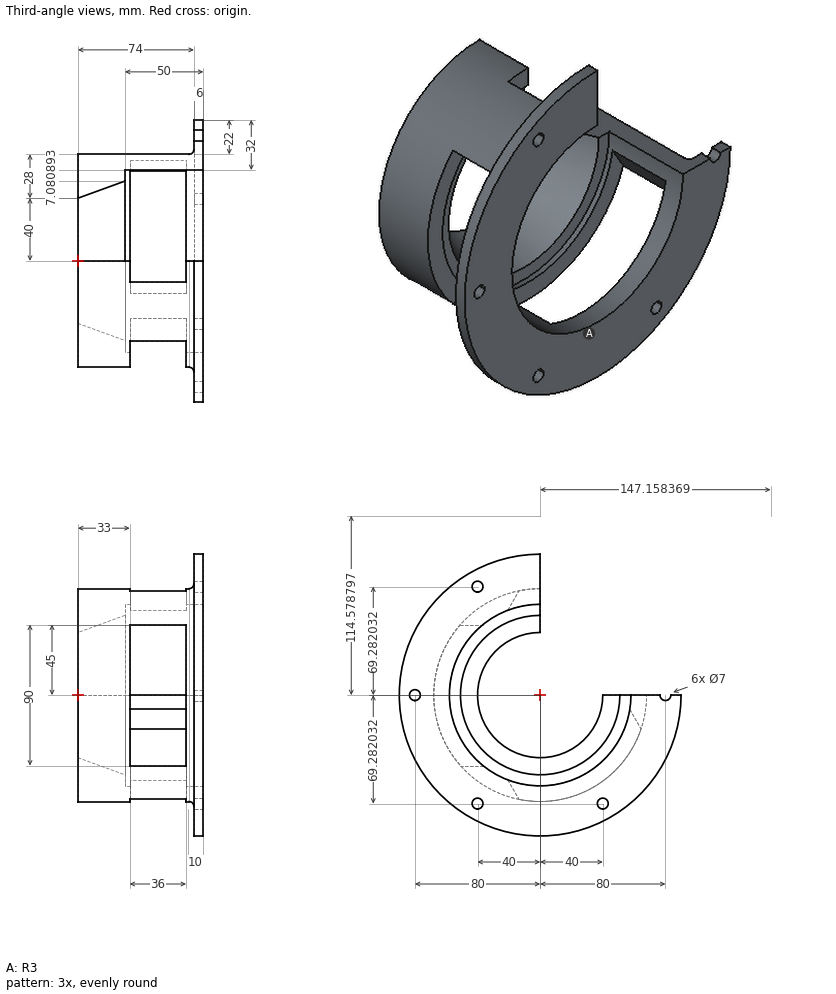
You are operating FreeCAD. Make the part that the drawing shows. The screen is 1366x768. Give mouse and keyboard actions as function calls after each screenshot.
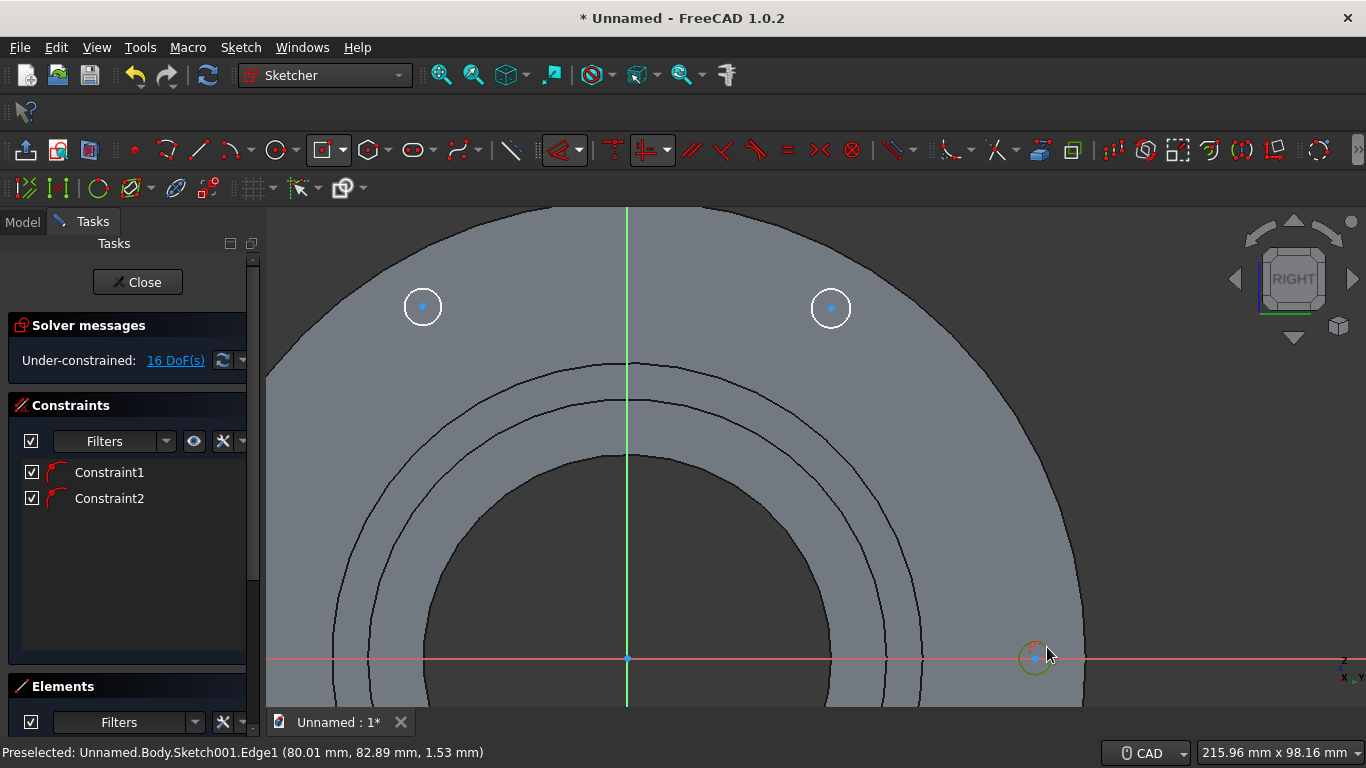
scroll(846, 293, down, 4)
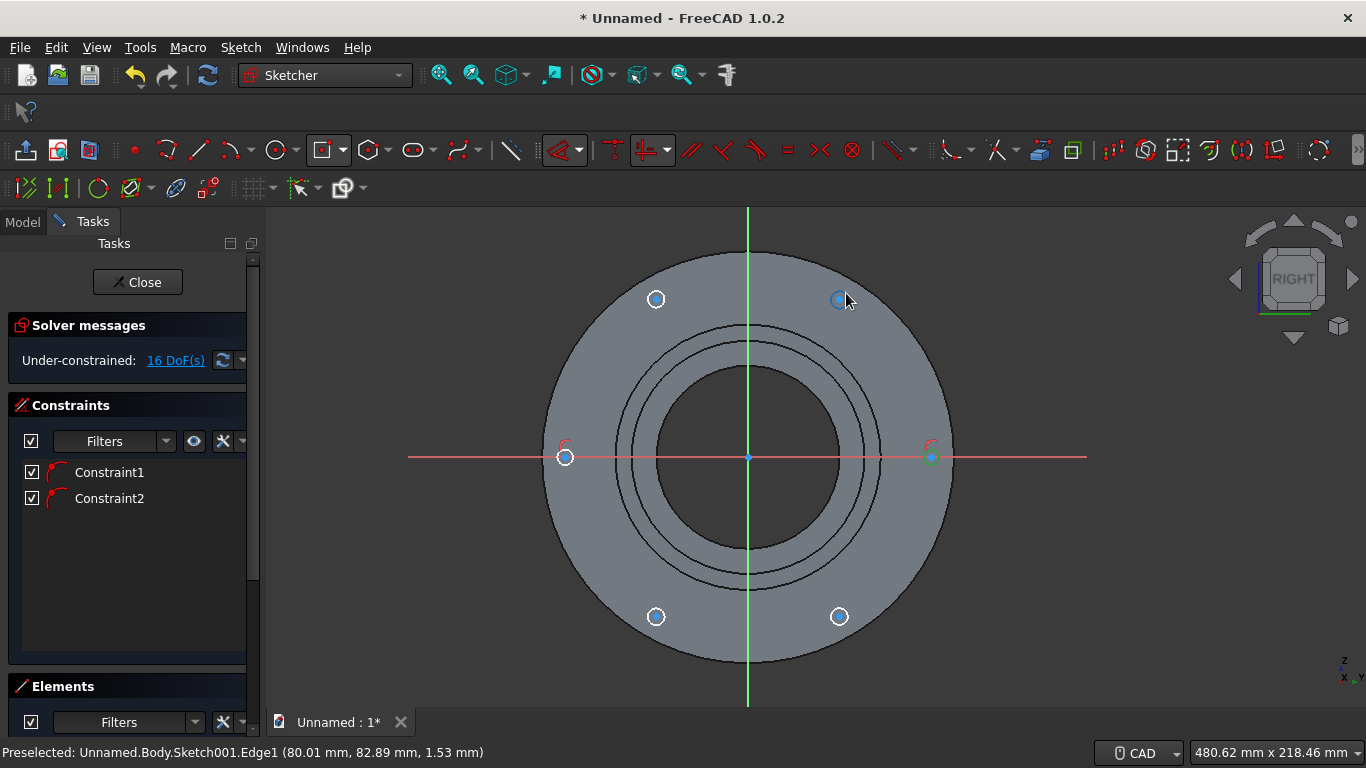
scroll(845, 611, up, 3)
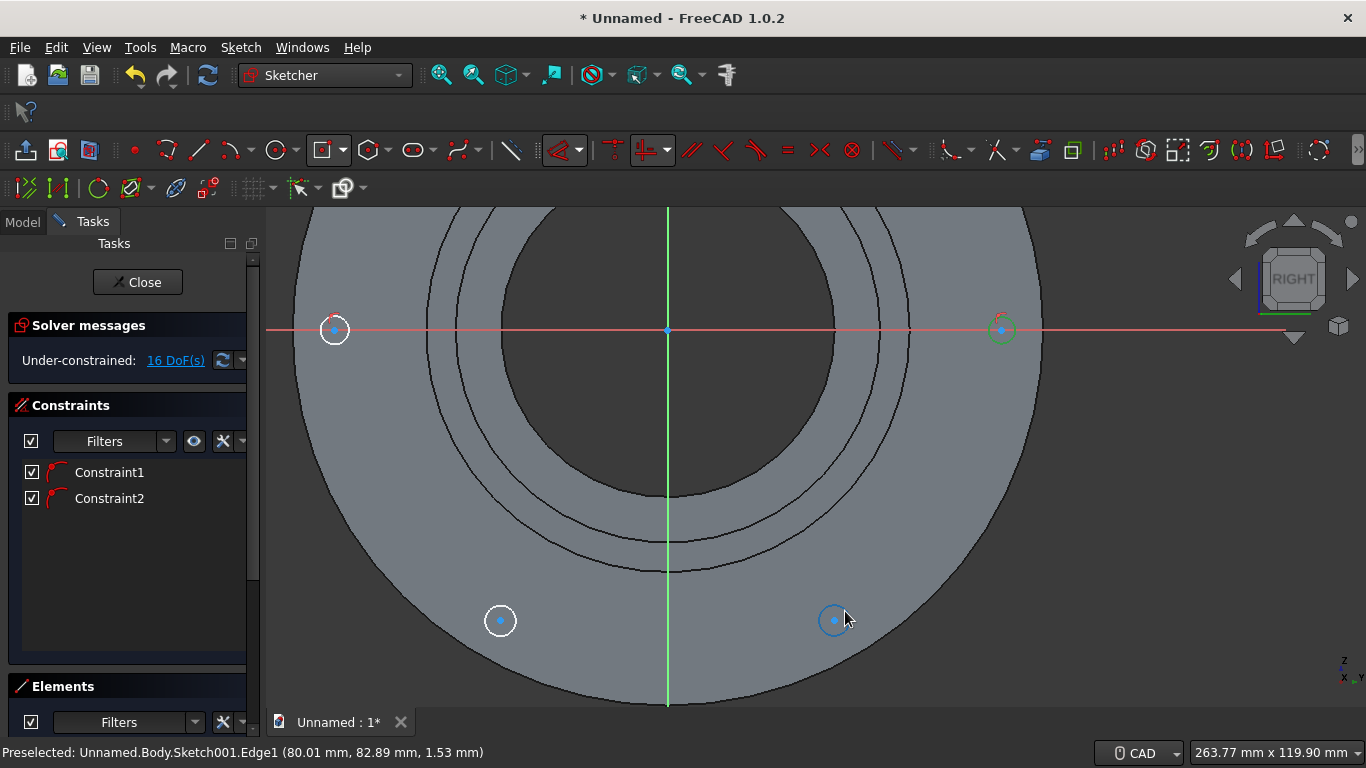
click(845, 610)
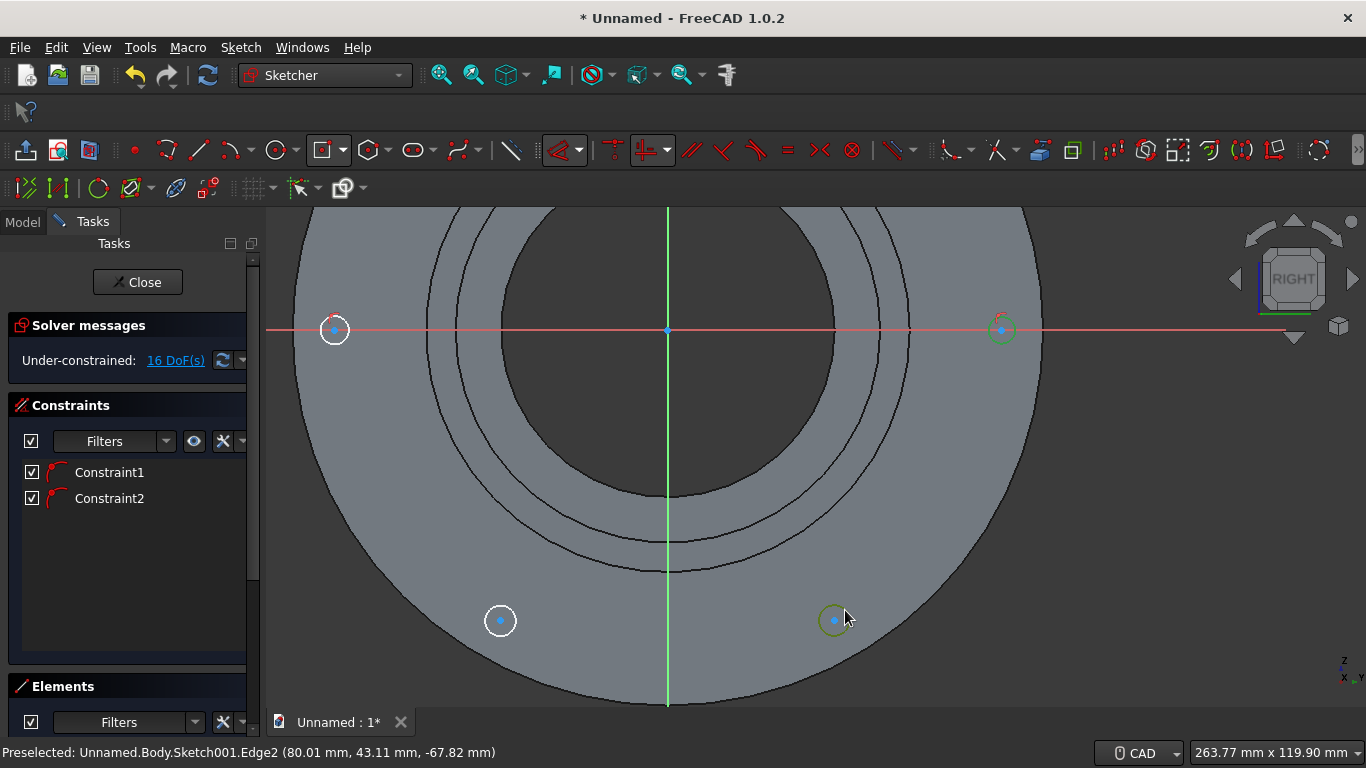
click(511, 610)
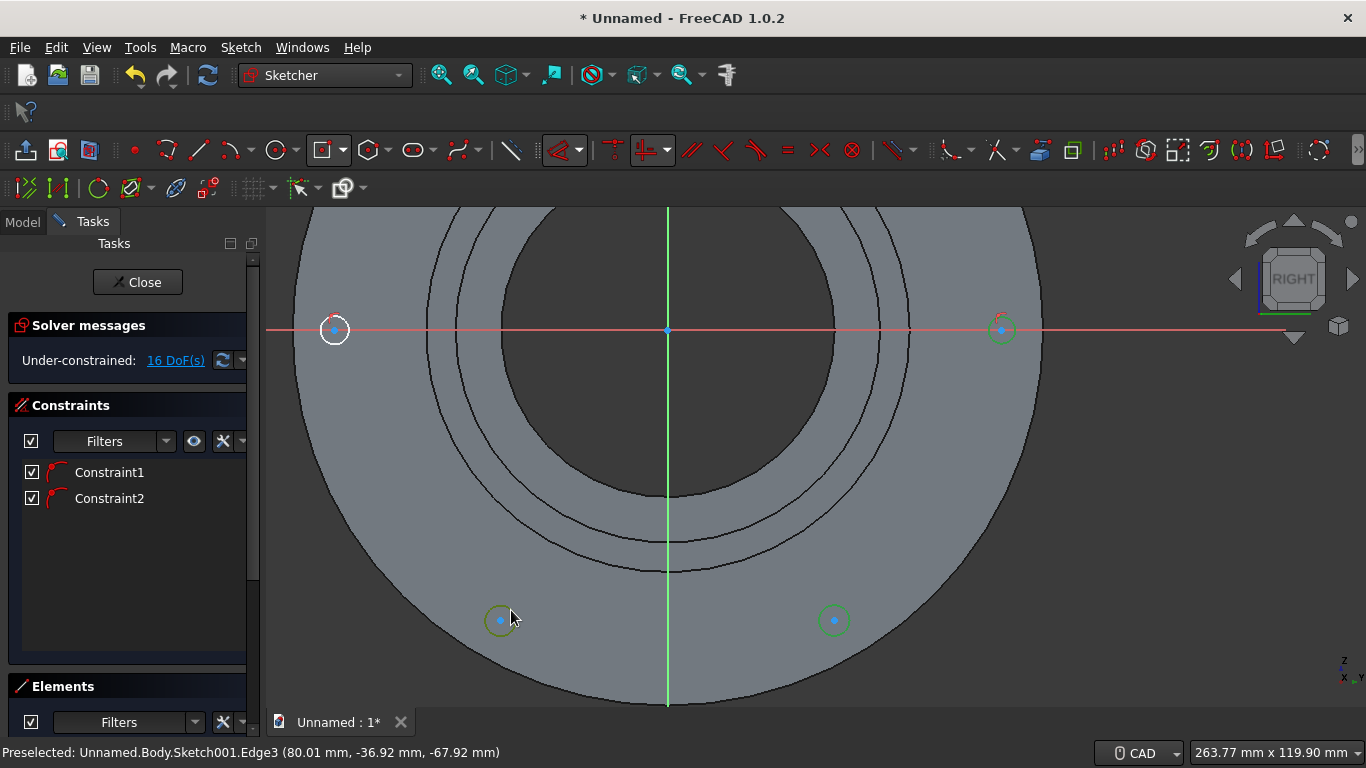
scroll(345, 320, up, 2)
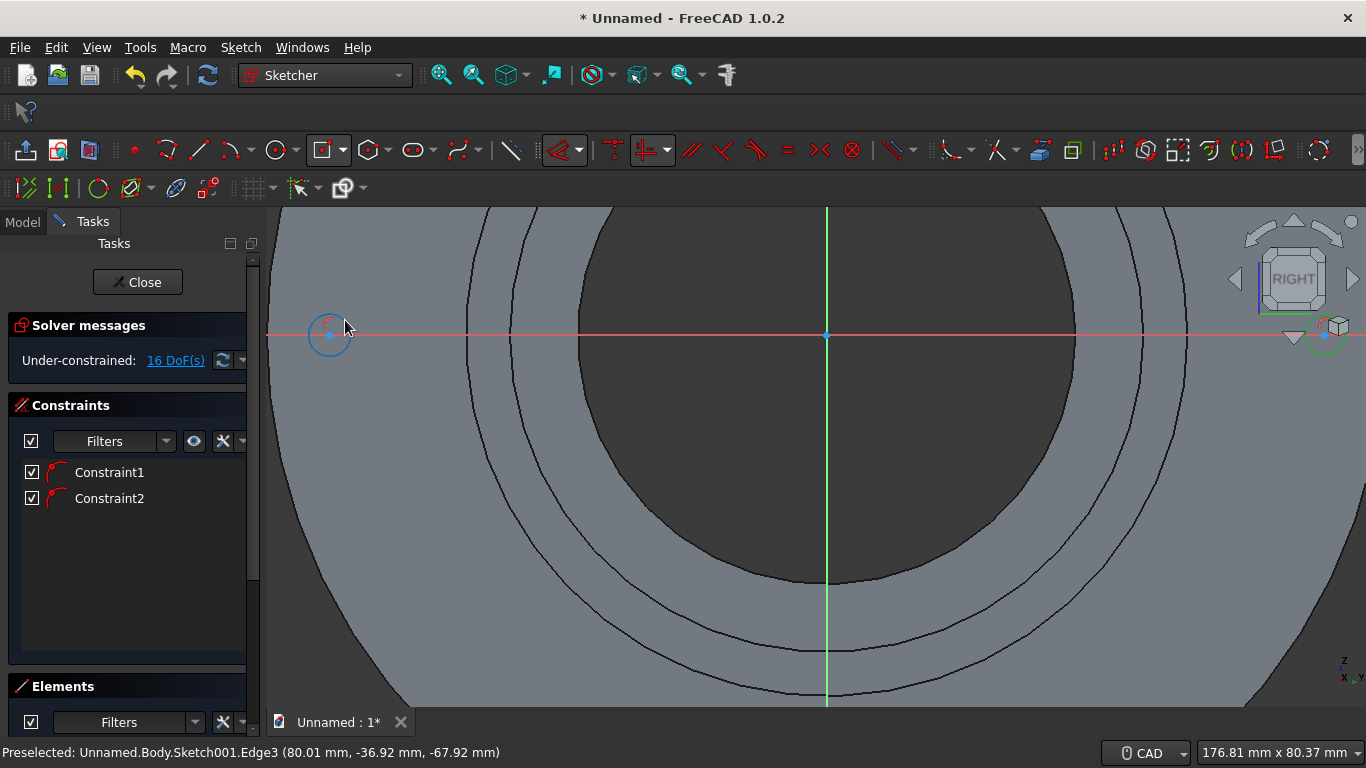
click(344, 320)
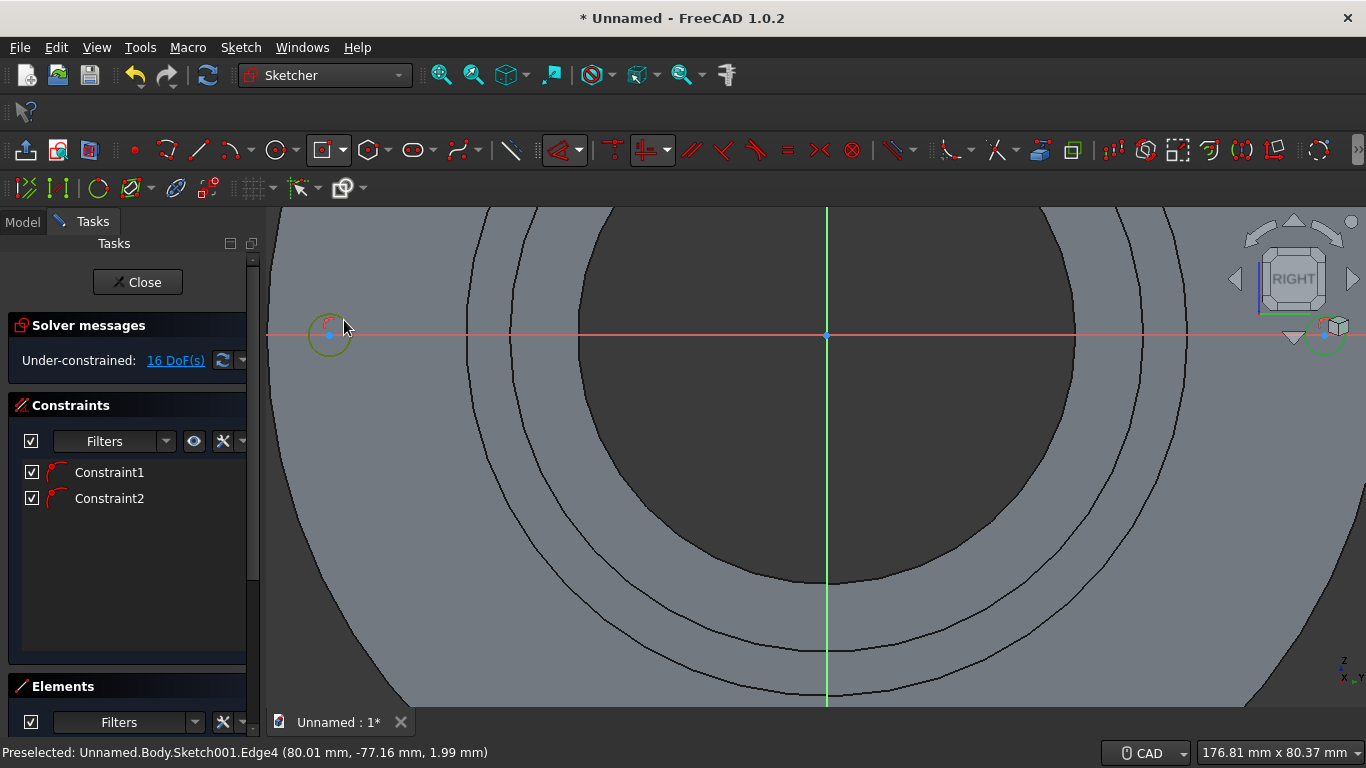
scroll(701, 528, down, 5)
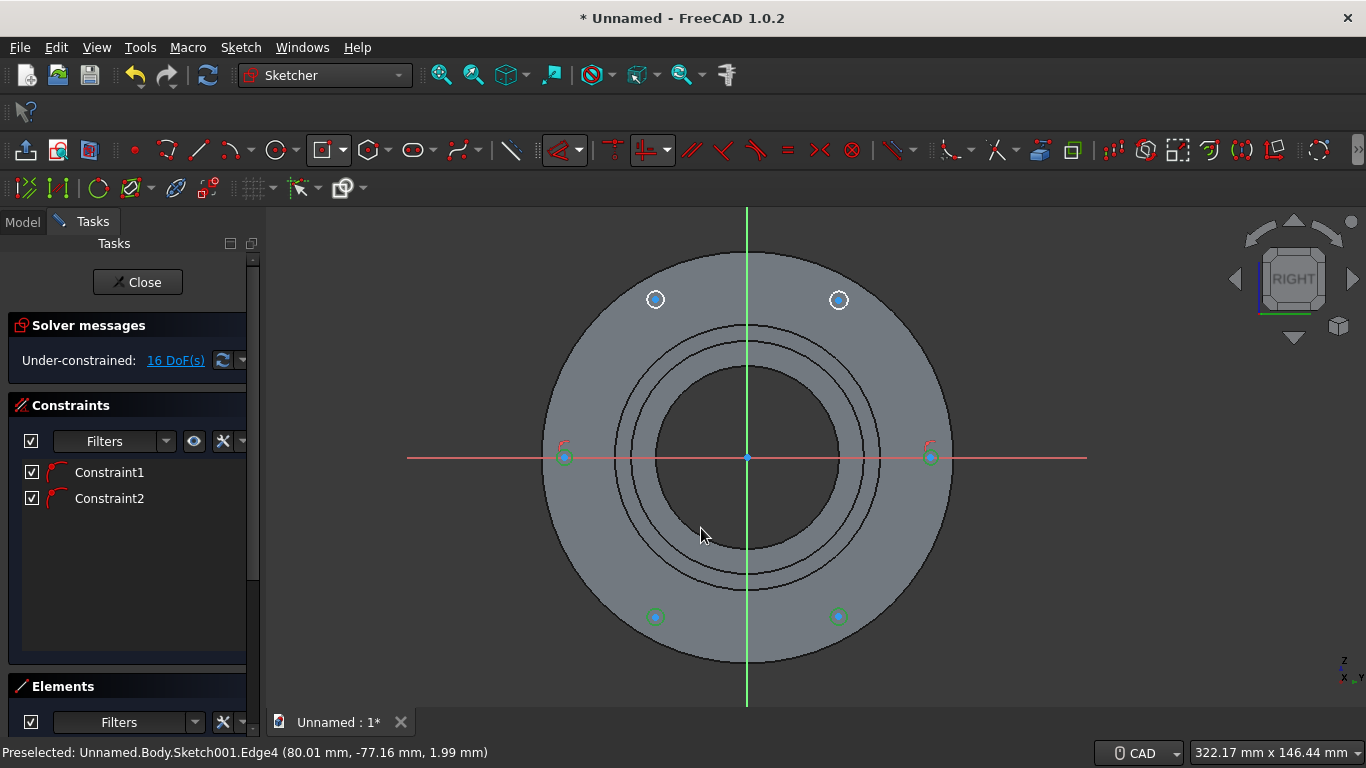
scroll(661, 294, up, 3)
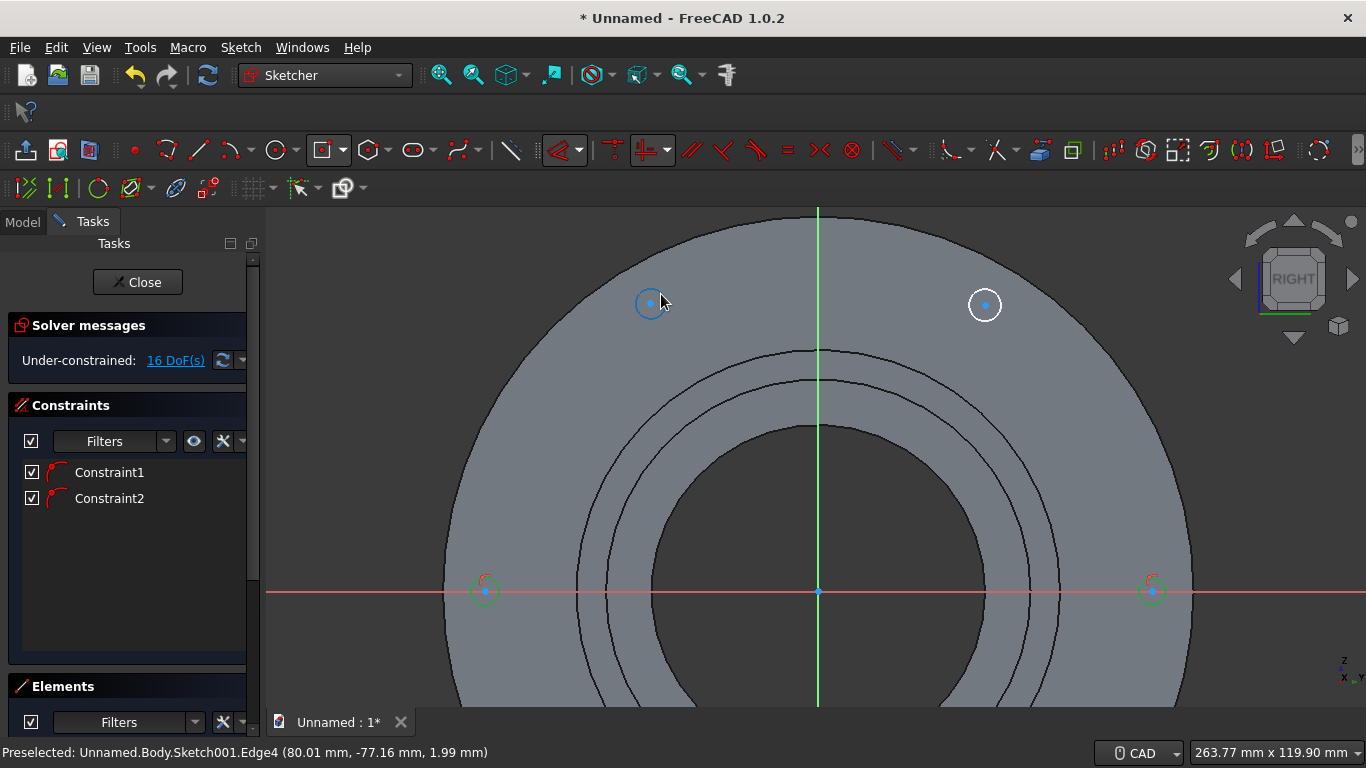
click(661, 293)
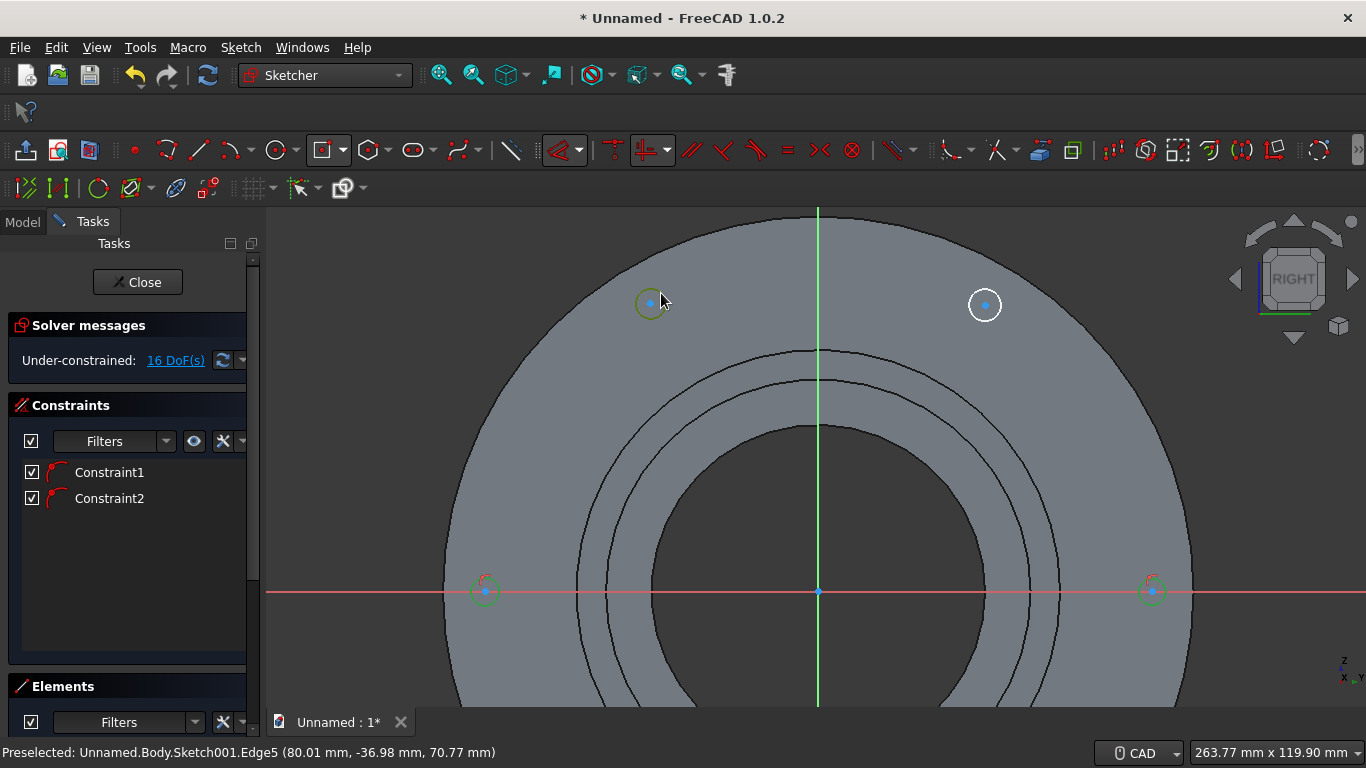
click(996, 294)